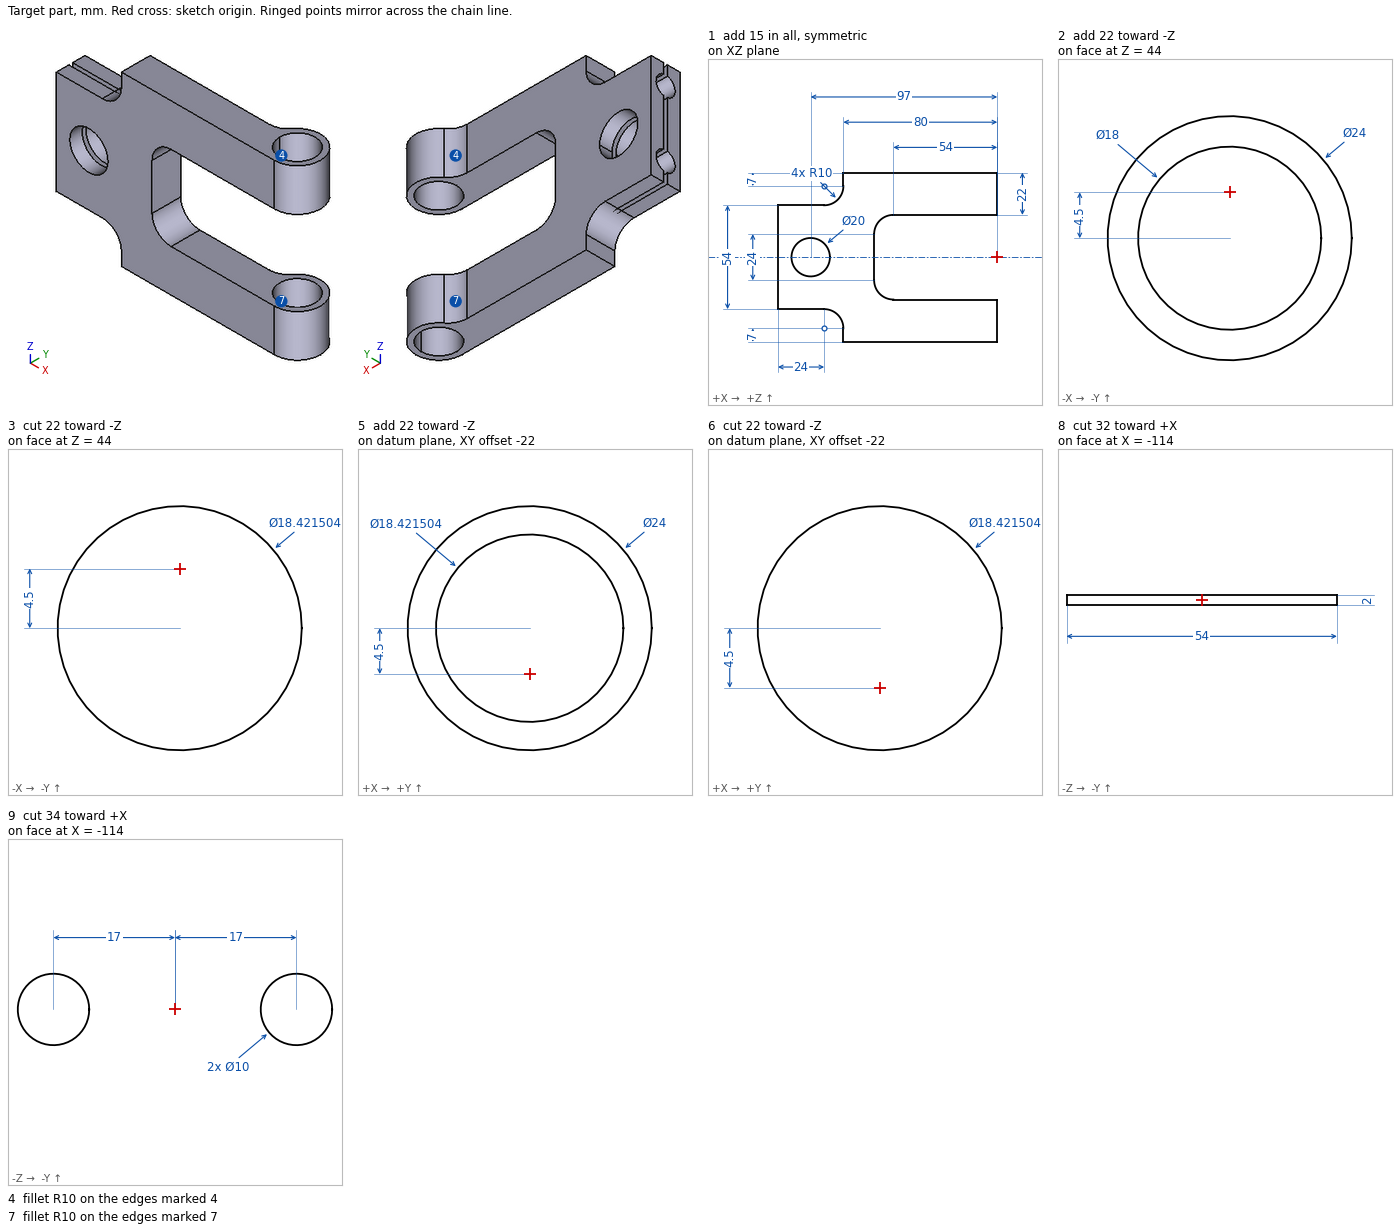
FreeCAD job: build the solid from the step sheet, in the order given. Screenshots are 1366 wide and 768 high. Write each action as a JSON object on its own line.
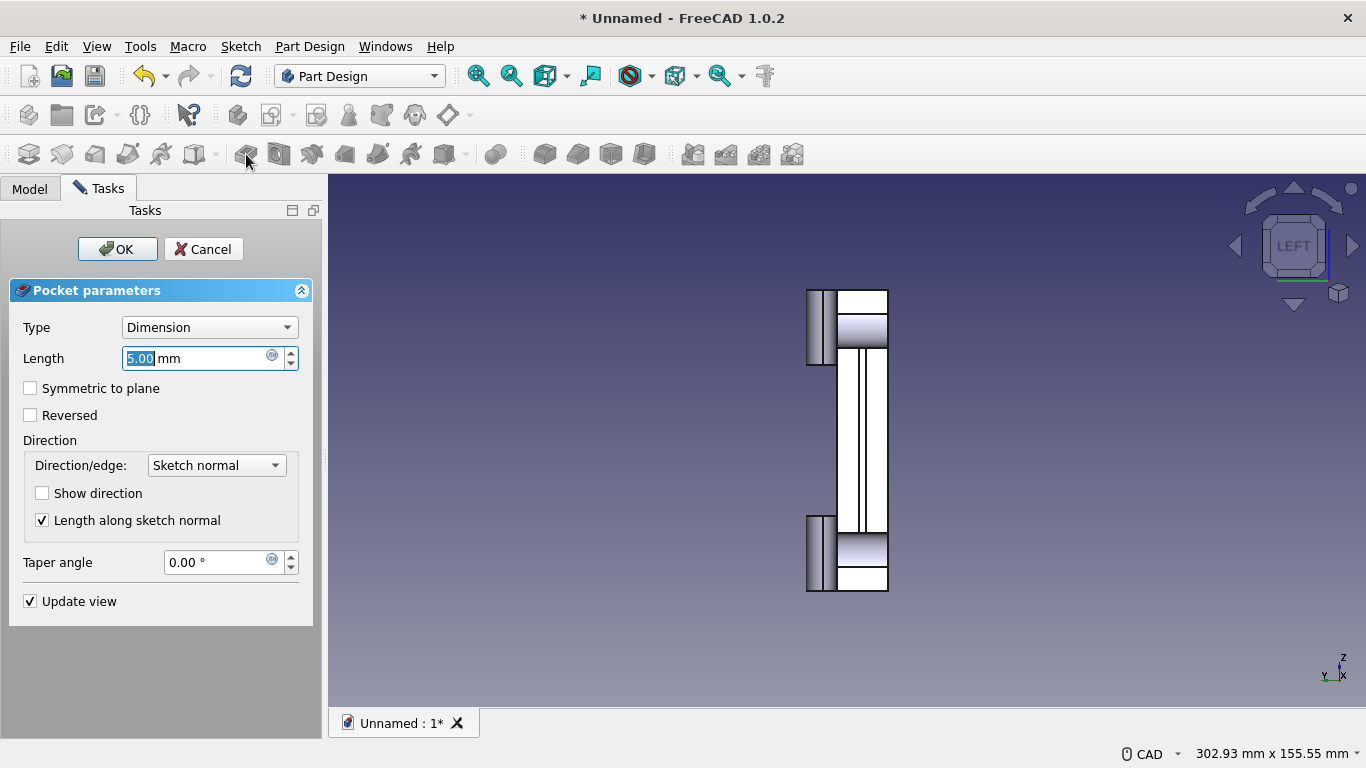
{"action": "type", "text": "32"}
{"action": "key", "text": "Tab"}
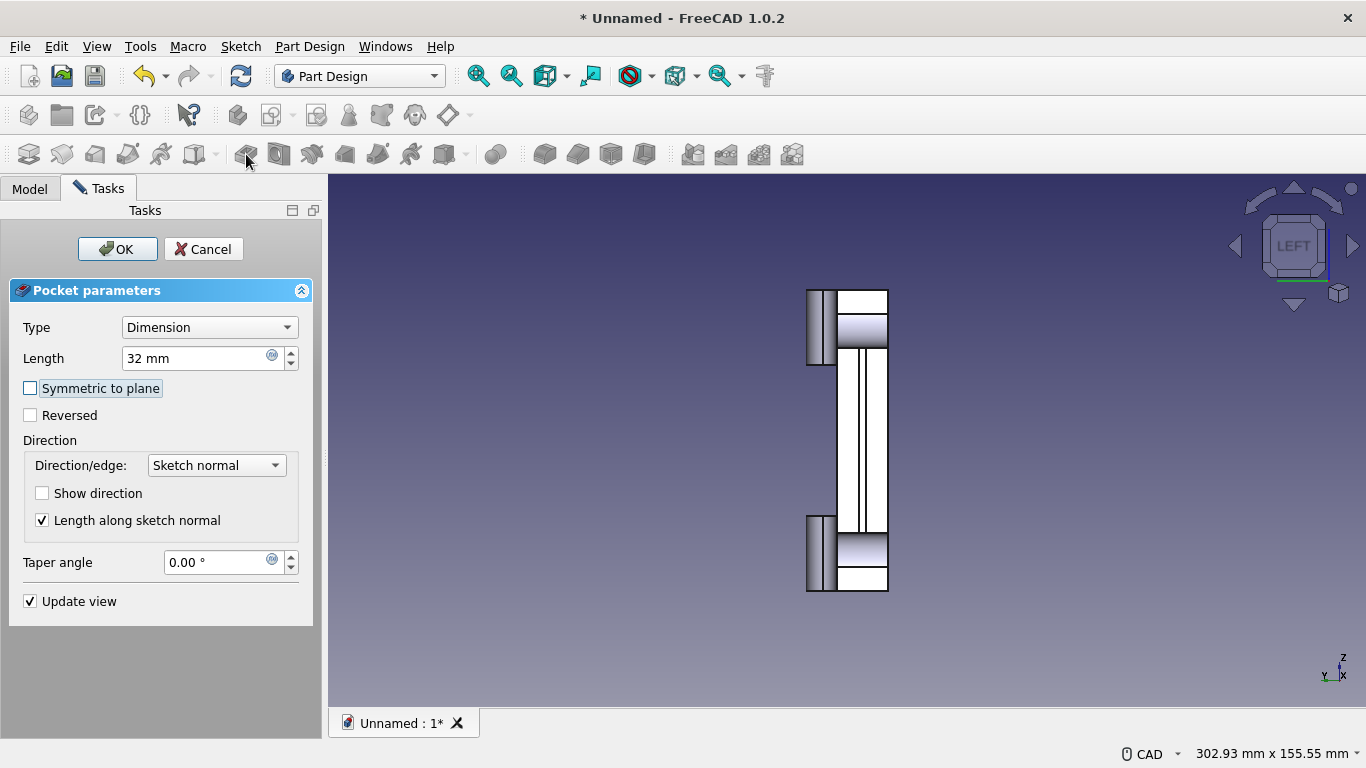
{"action": "left_click", "coordinate": [118, 249]}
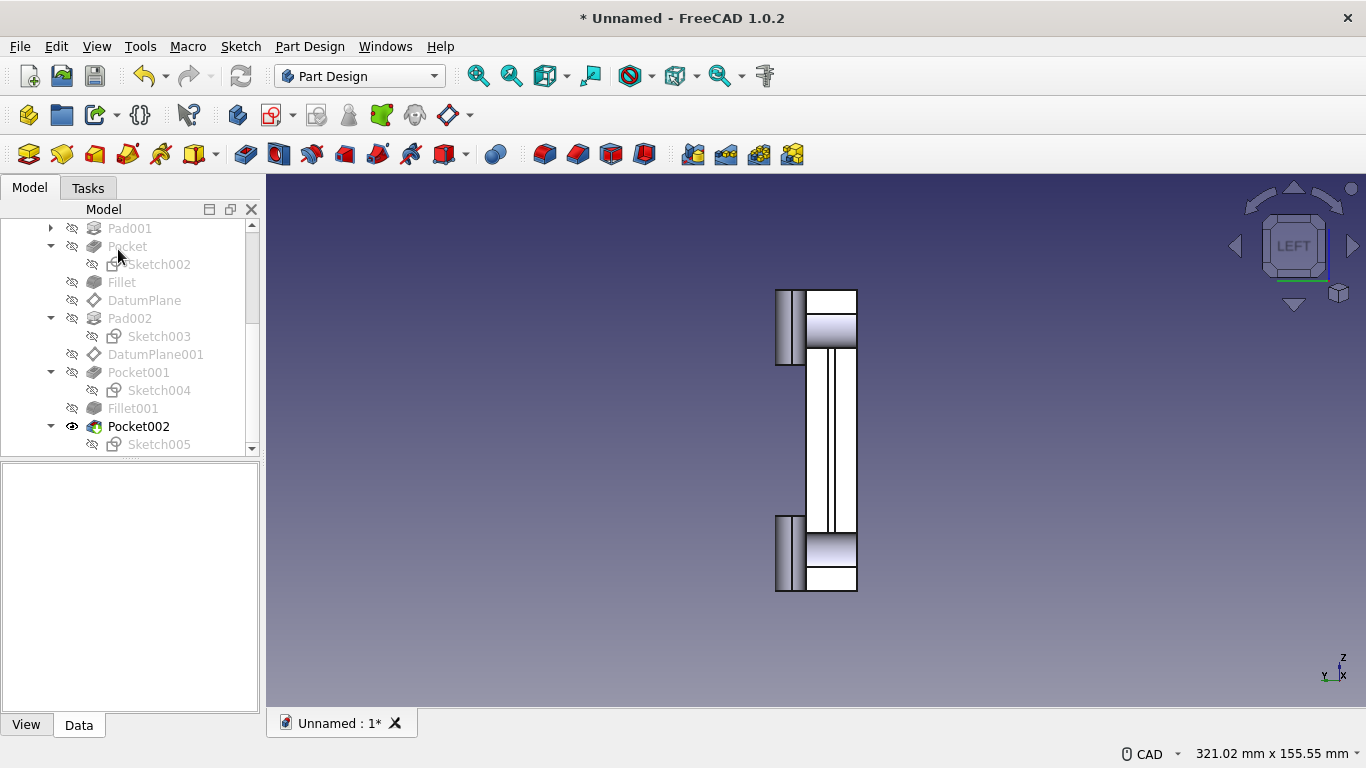
{"action": "left_click", "coordinate": [817, 360]}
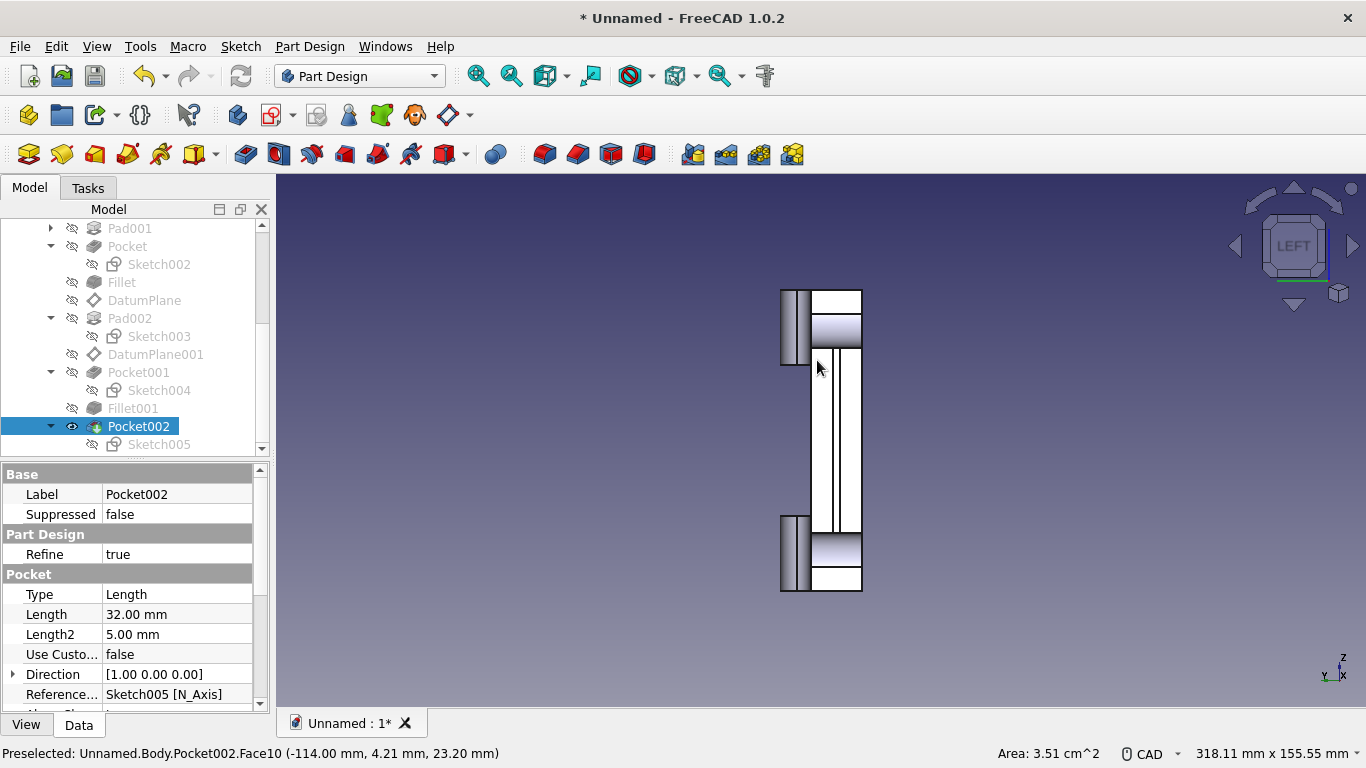
{"action": "left_click", "coordinate": [270, 116]}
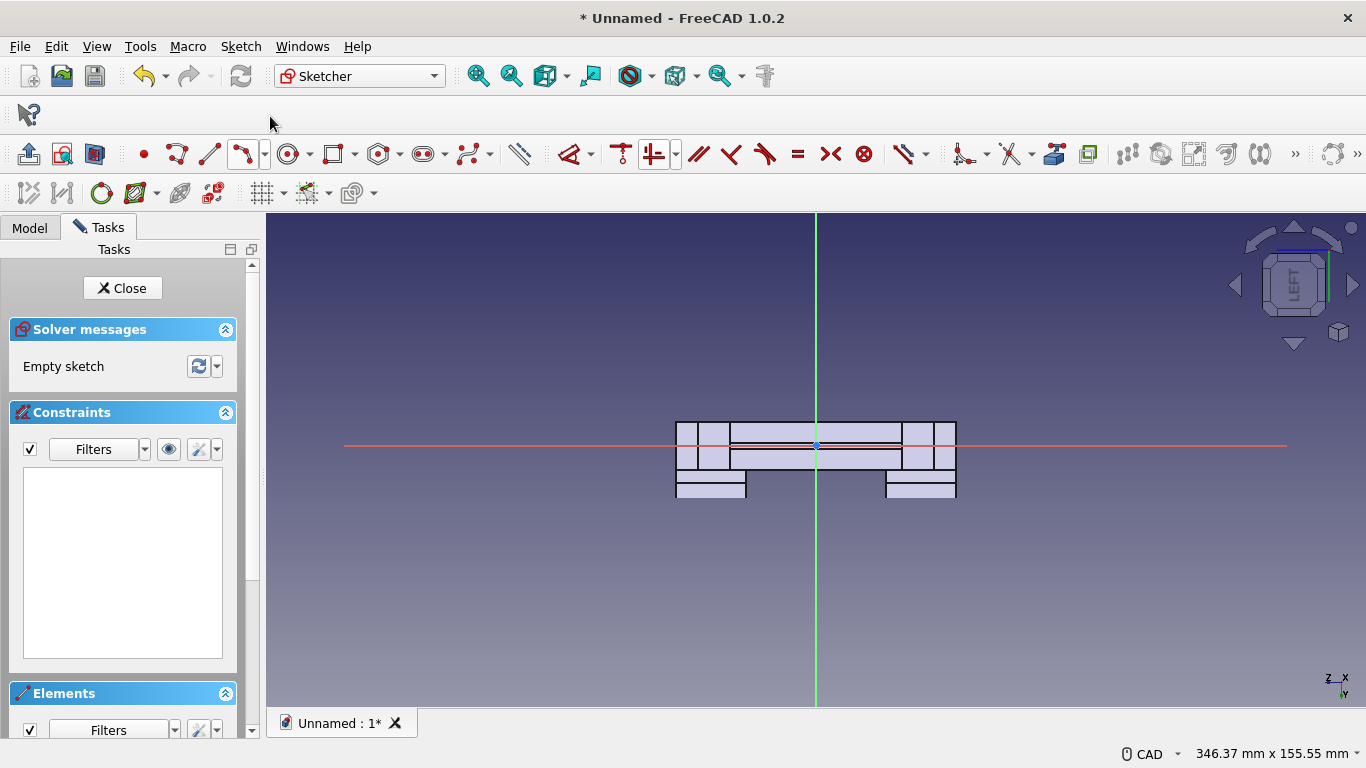
{"action": "scroll", "coordinate": [833, 442], "scroll_direction": "up", "scroll_amount": 8}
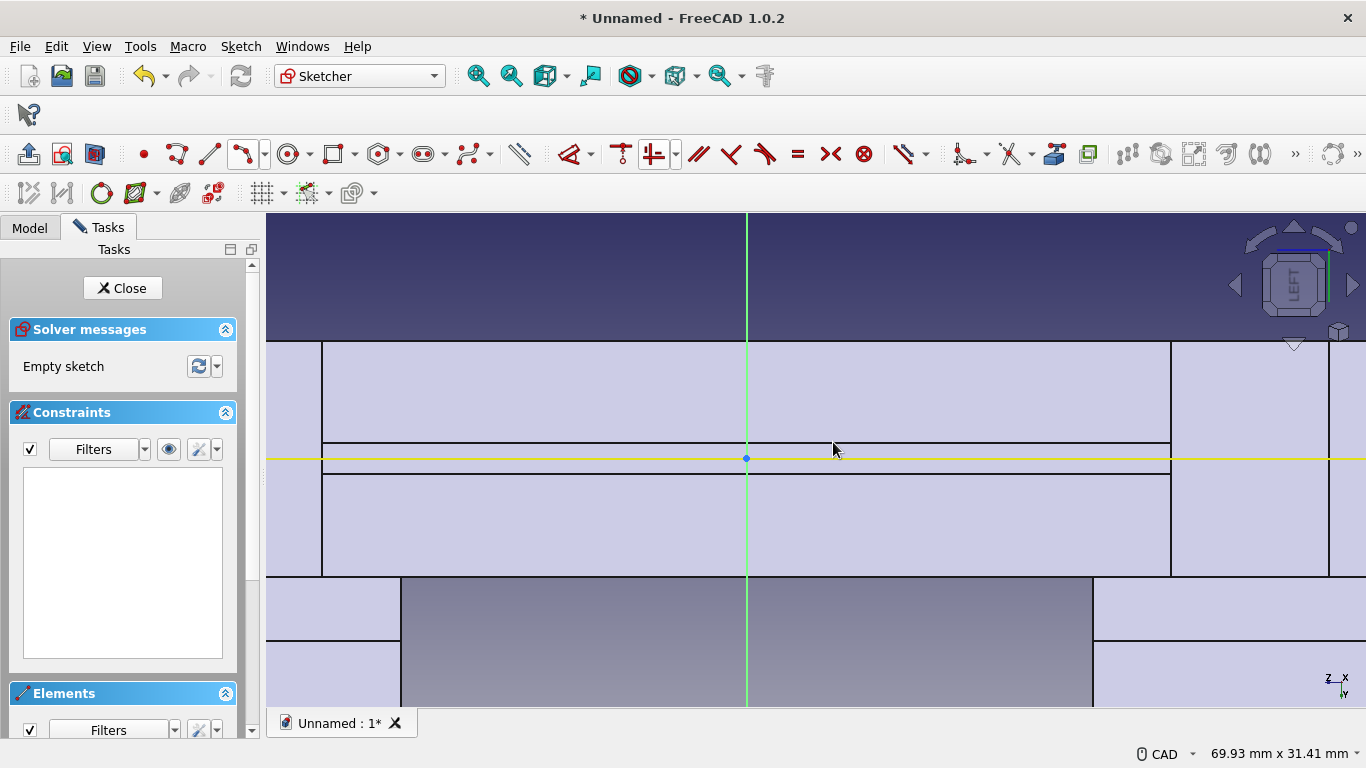
{"action": "left_click", "coordinate": [288, 154]}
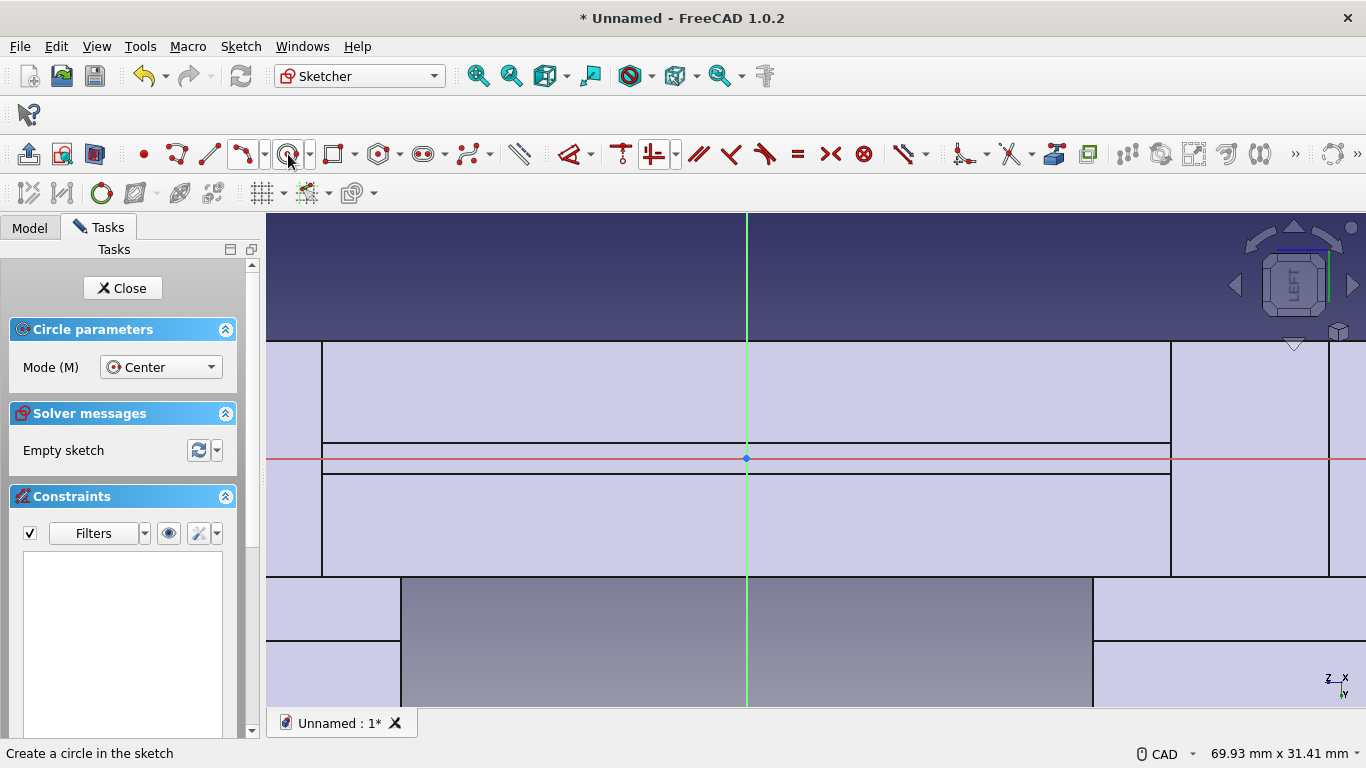
{"action": "left_click", "coordinate": [1014, 459]}
{"action": "left_click", "coordinate": [1070, 403]}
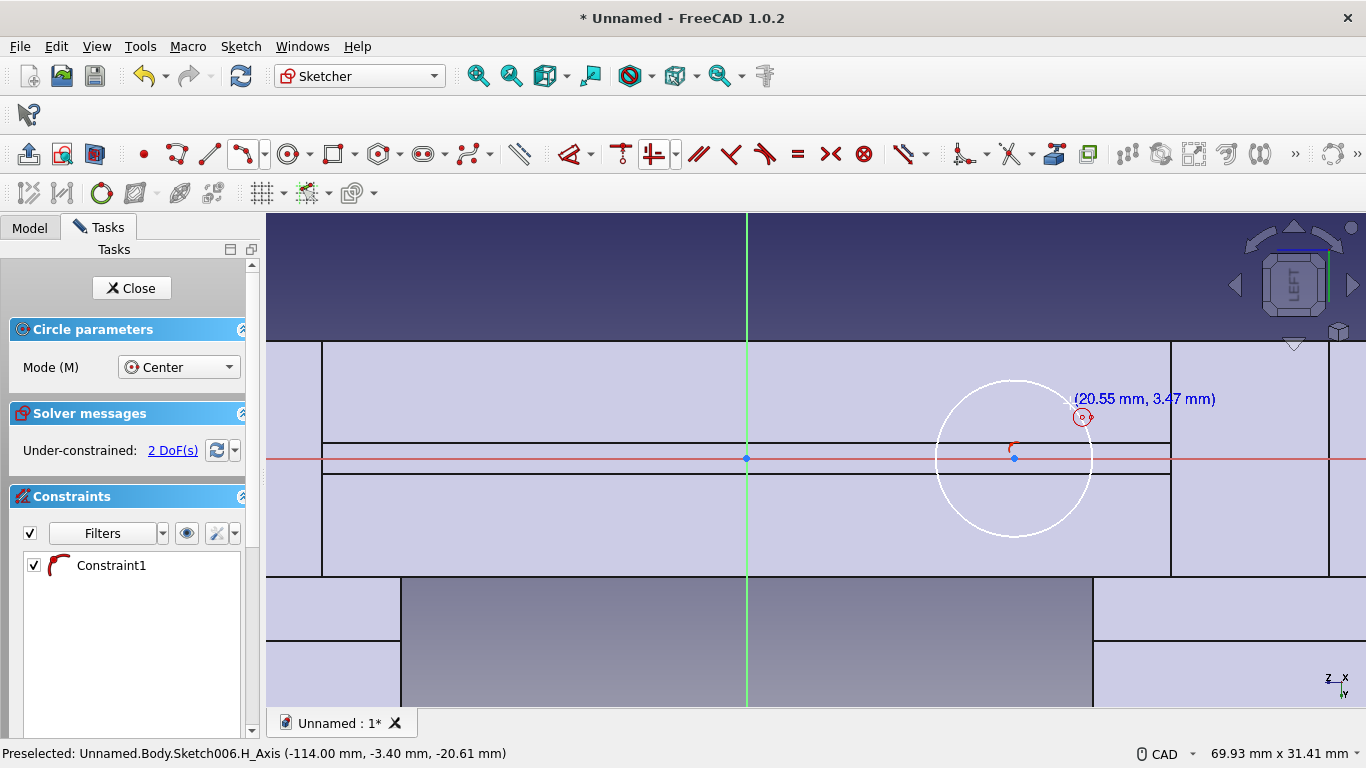
{"action": "left_click", "coordinate": [479, 459]}
{"action": "left_click", "coordinate": [535, 403]}
{"action": "key", "text": "Escape"}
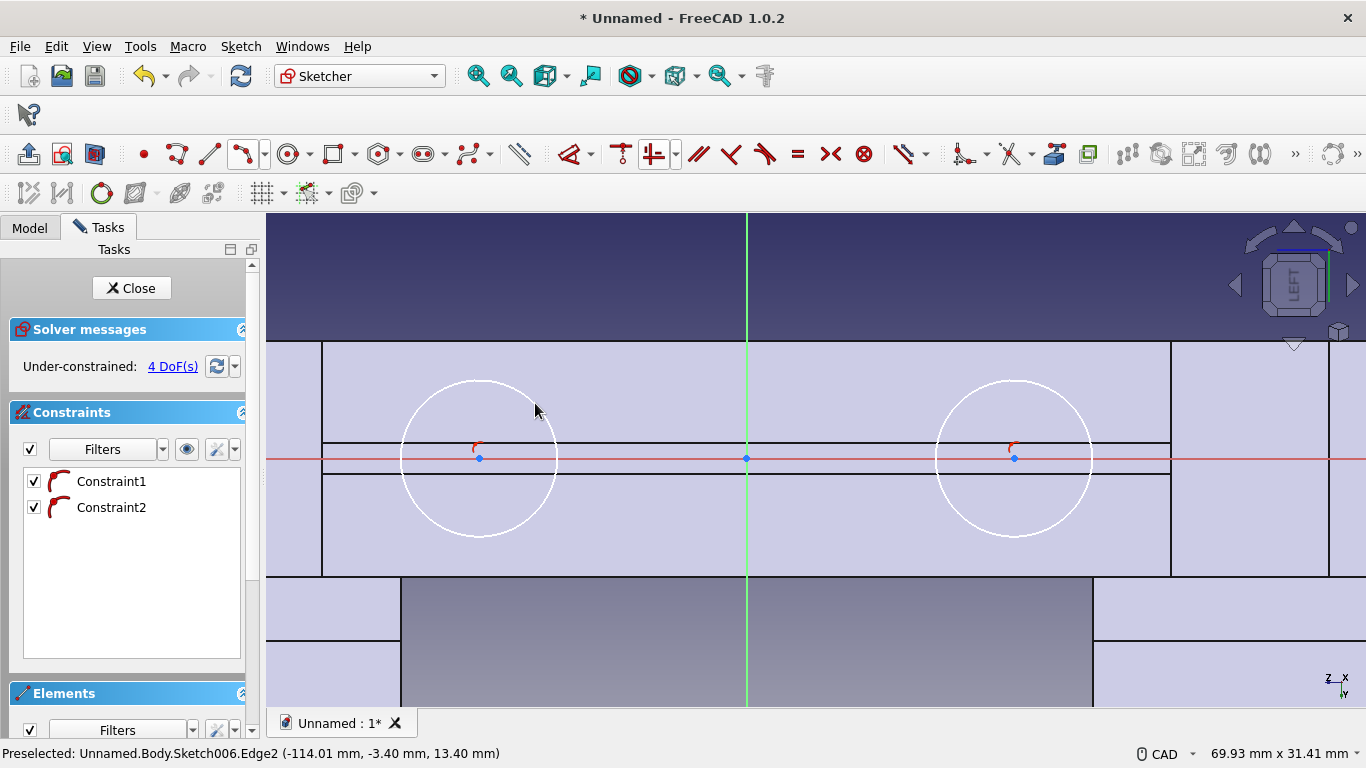
{"action": "left_click", "coordinate": [1069, 403]}